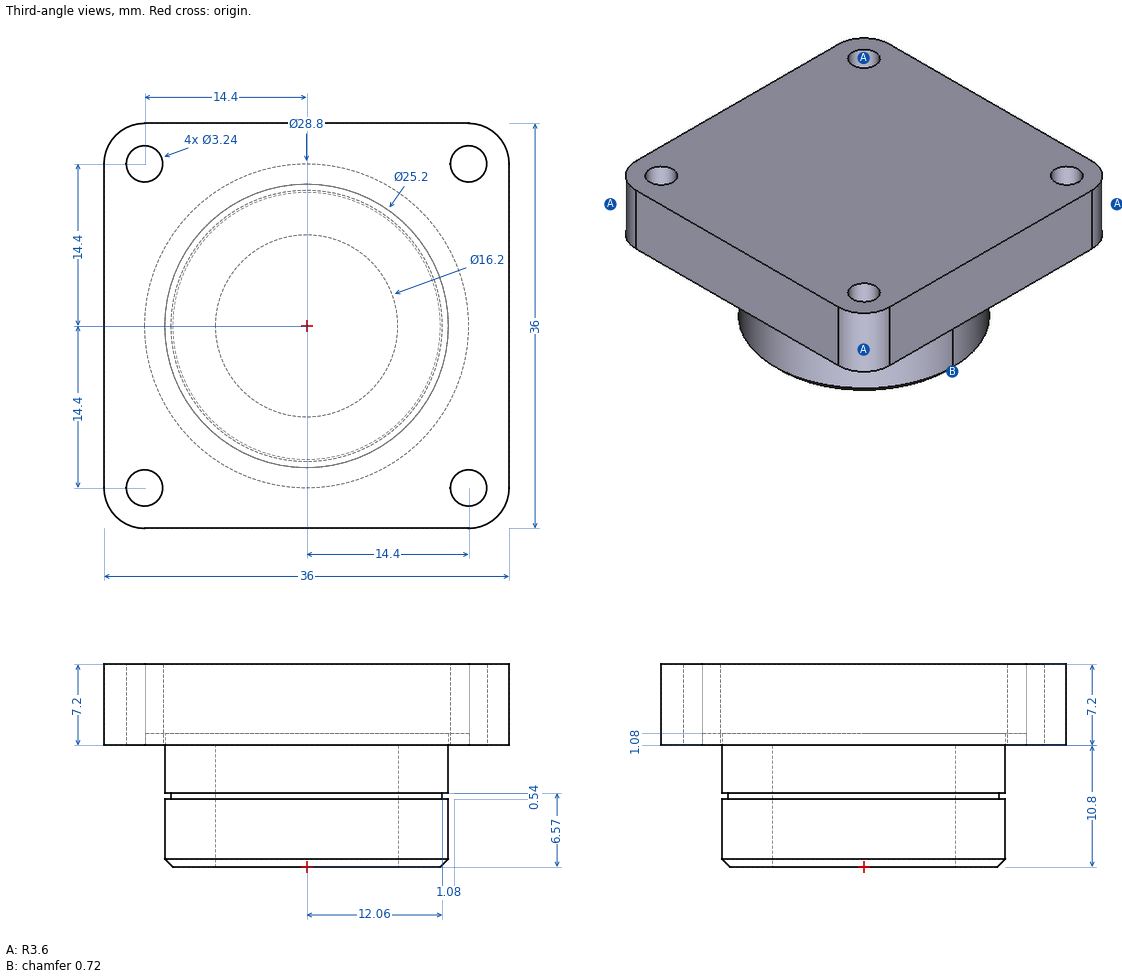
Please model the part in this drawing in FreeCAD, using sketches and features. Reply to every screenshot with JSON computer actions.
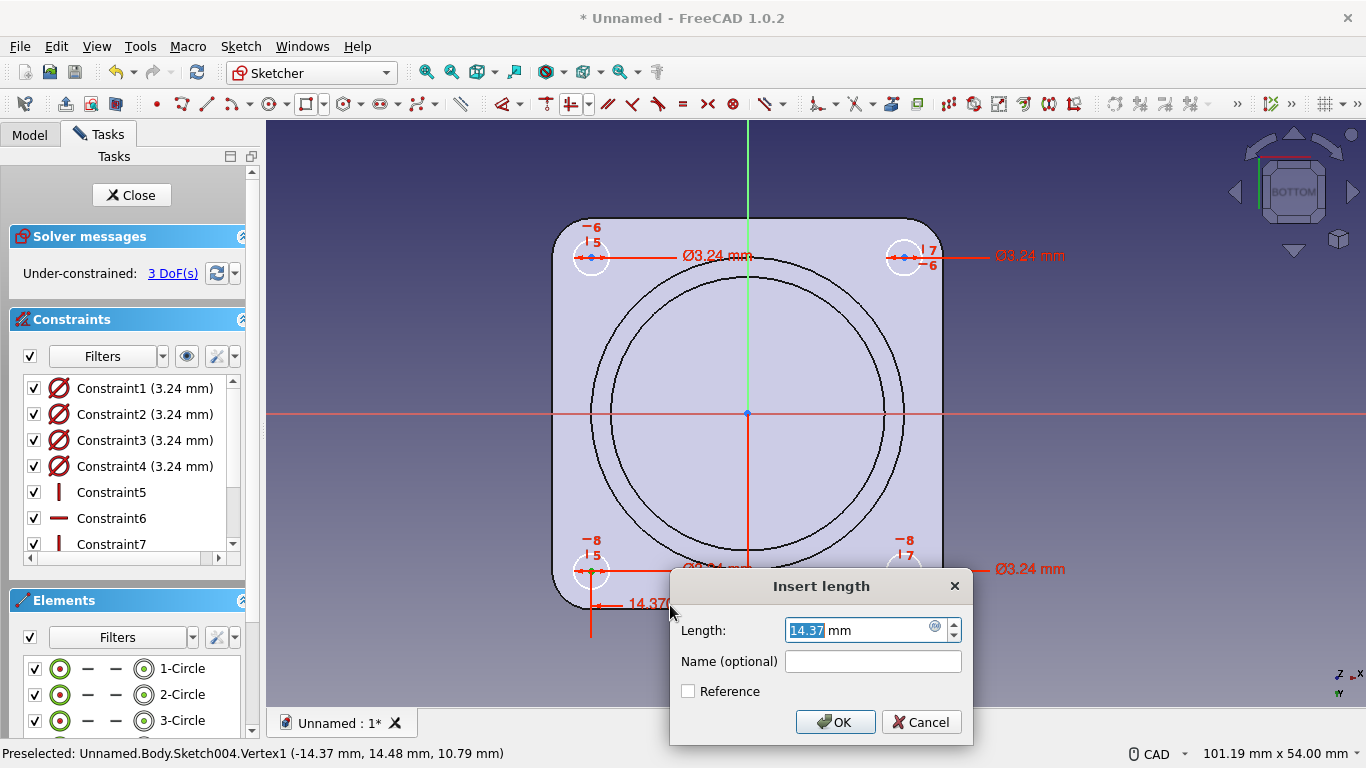
{"action": "type", "text": "14.4"}
{"action": "key", "text": "Return"}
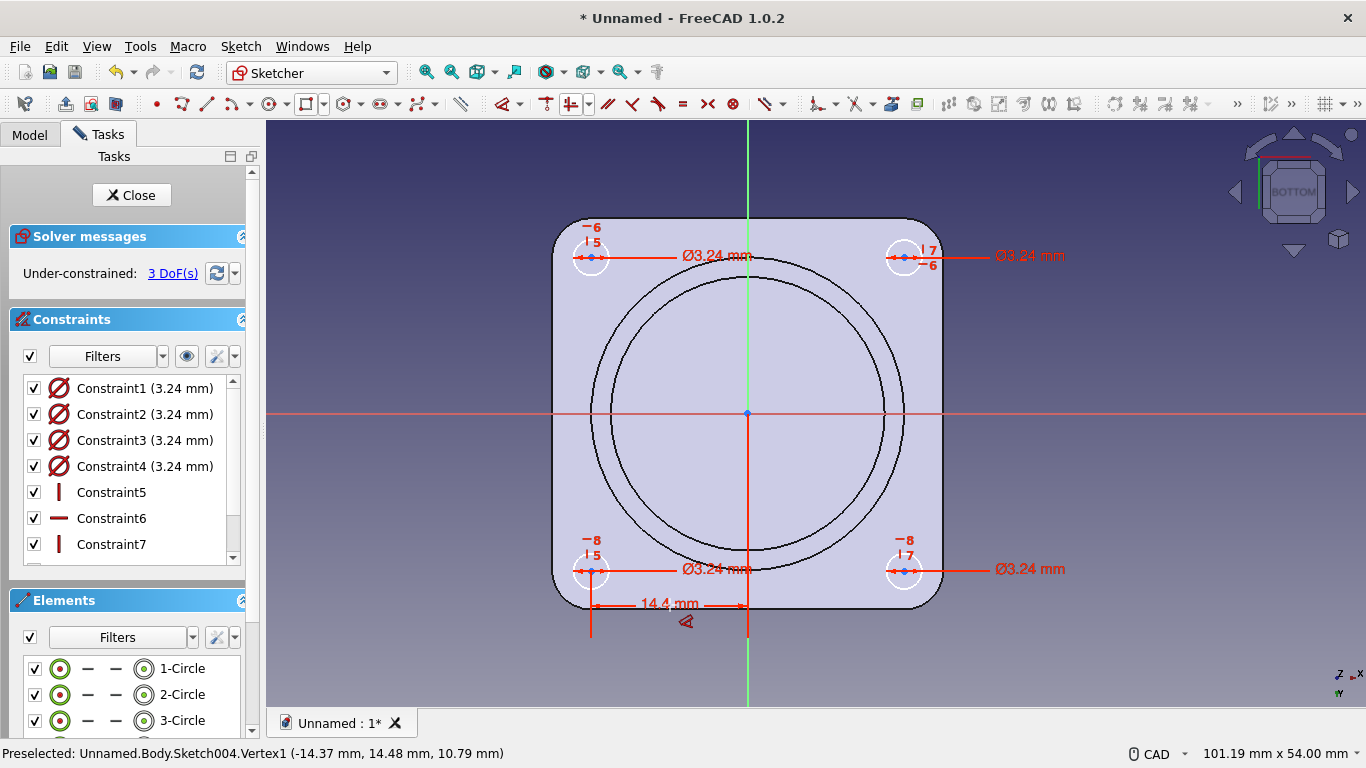
{"action": "left_click", "coordinate": [591, 571]}
{"action": "left_click", "coordinate": [557, 493]}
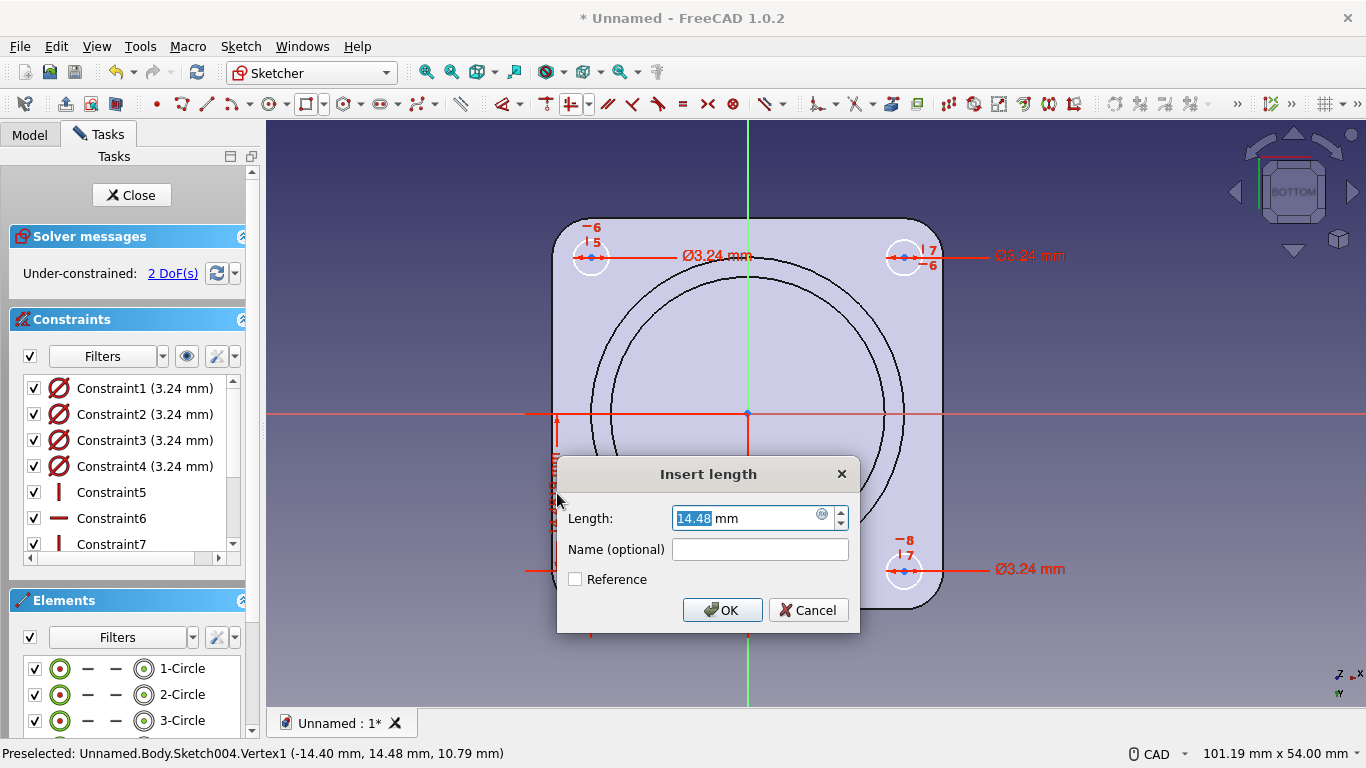
{"action": "type", "text": "14.4"}
{"action": "key", "text": "Return"}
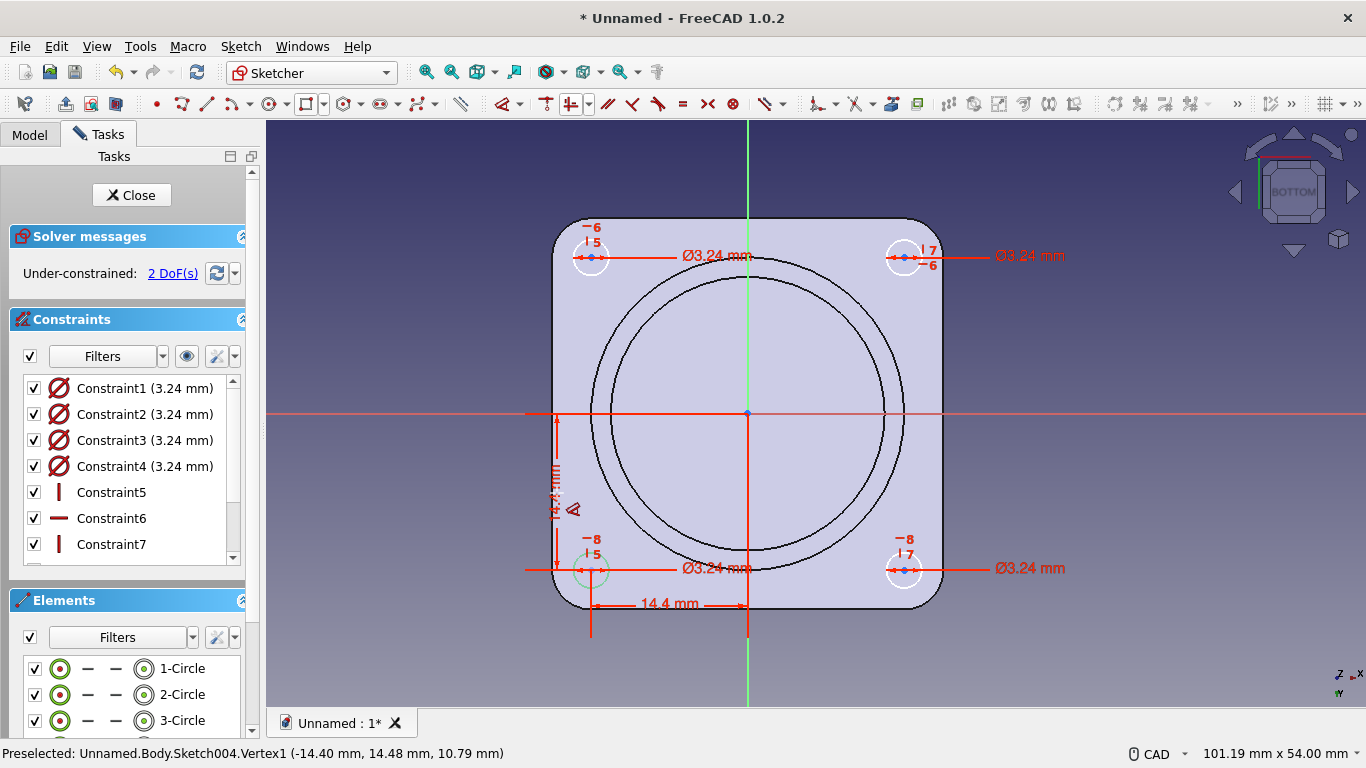
{"action": "left_click", "coordinate": [591, 258]}
{"action": "left_click", "coordinate": [557, 336]}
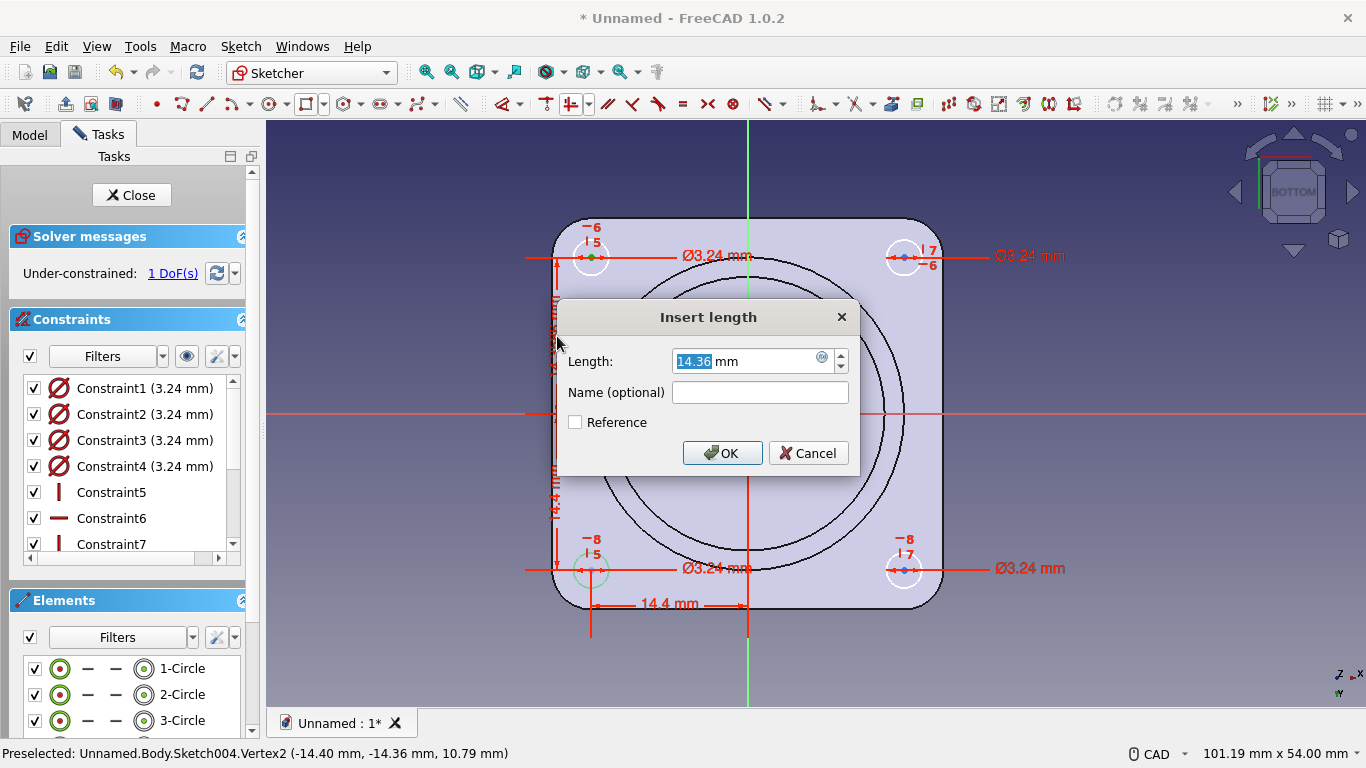
{"action": "type", "text": "14.4"}
{"action": "key", "text": "Return"}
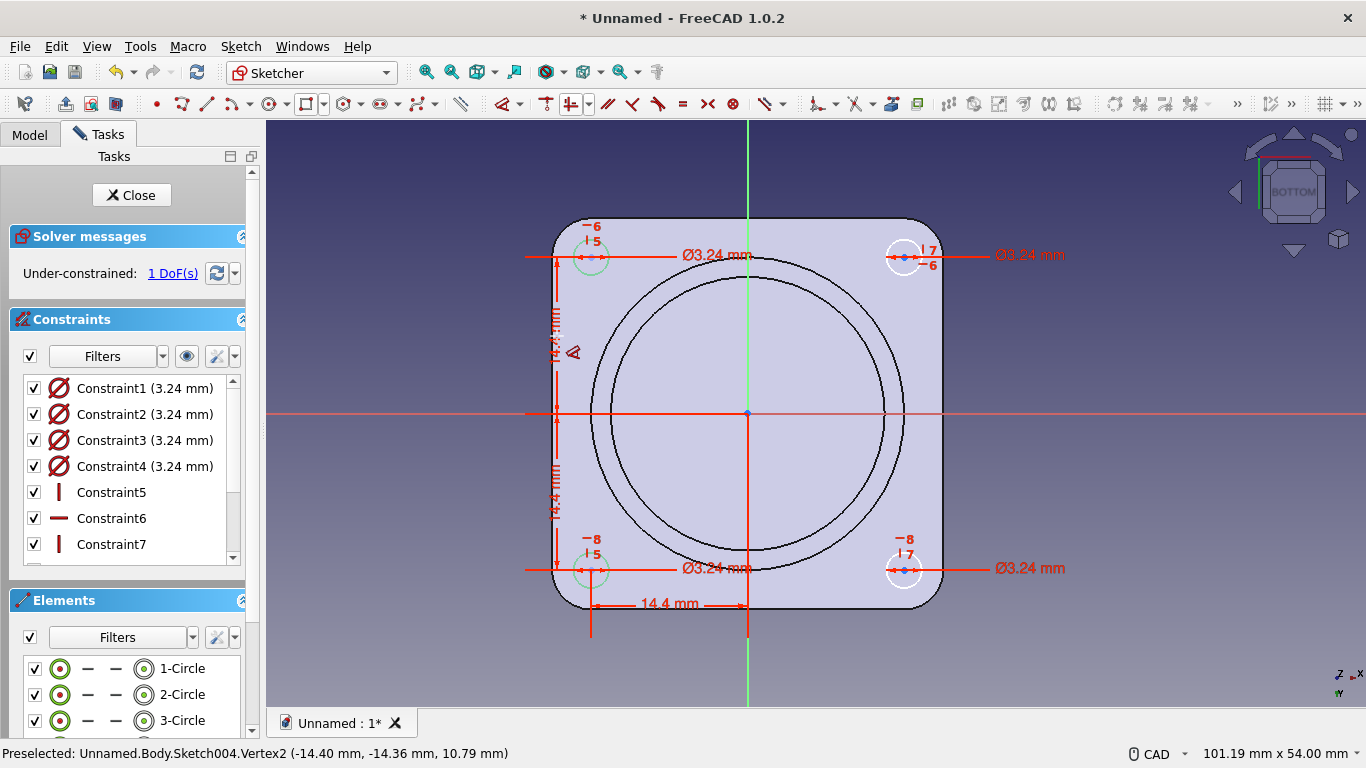
{"action": "left_click", "coordinate": [904, 257]}
{"action": "left_click", "coordinate": [826, 223]}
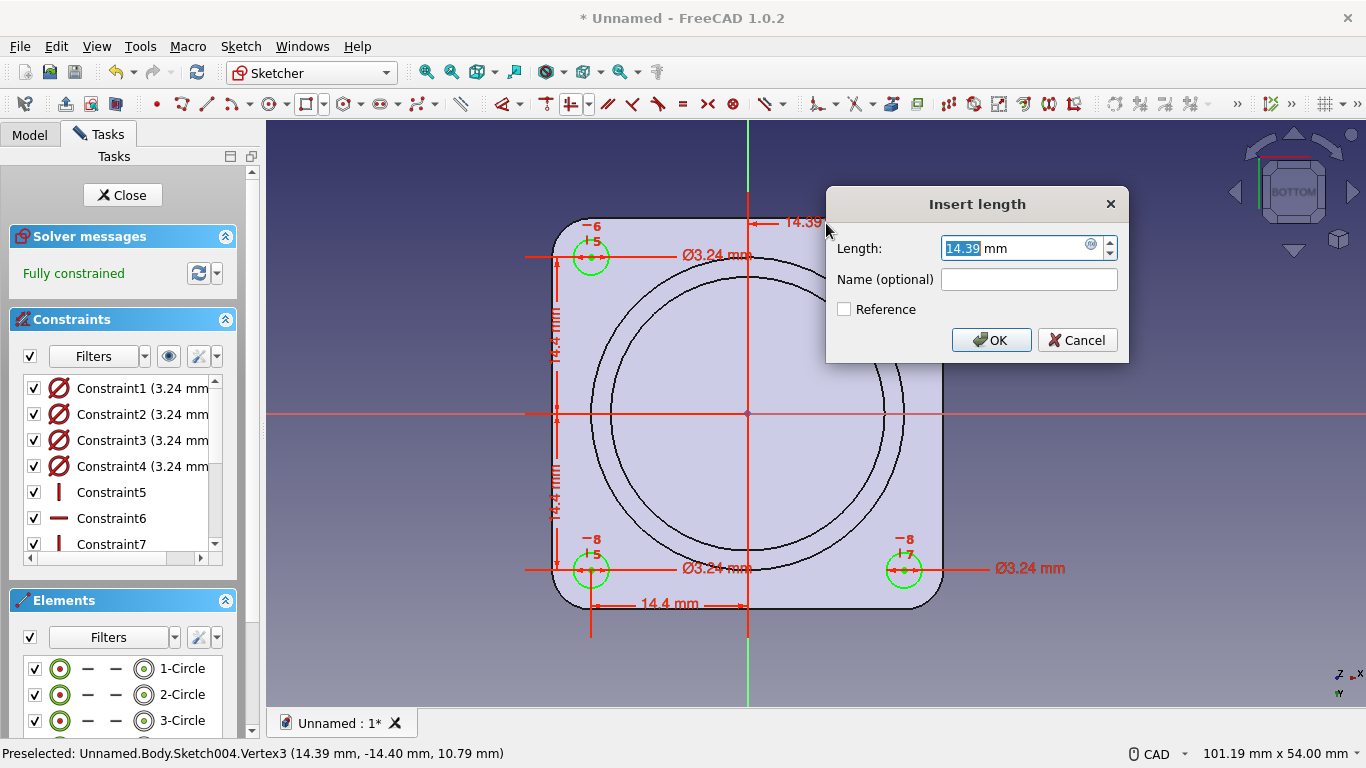
{"action": "type", "text": "14.4"}
{"action": "key", "text": "Return"}
{"action": "key", "text": "Escape"}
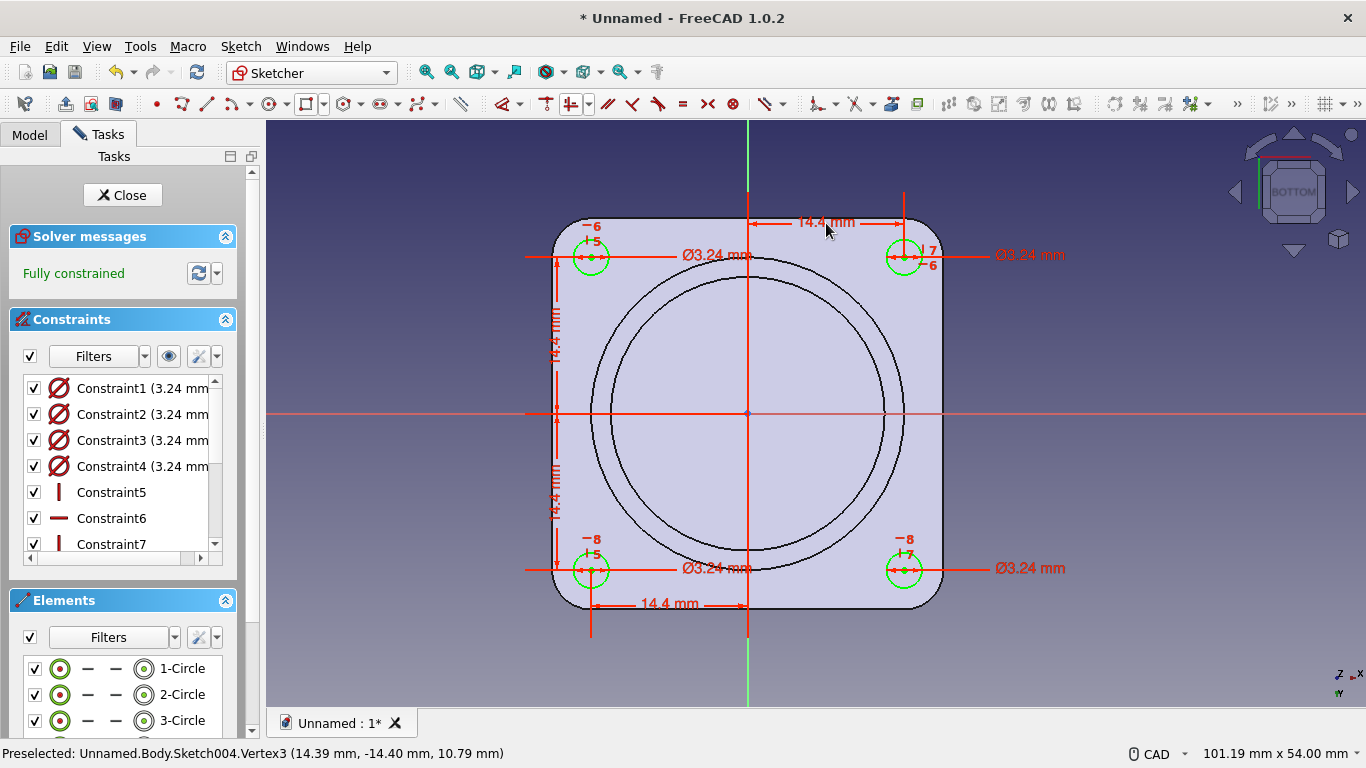
{"action": "left_click", "coordinate": [123, 195]}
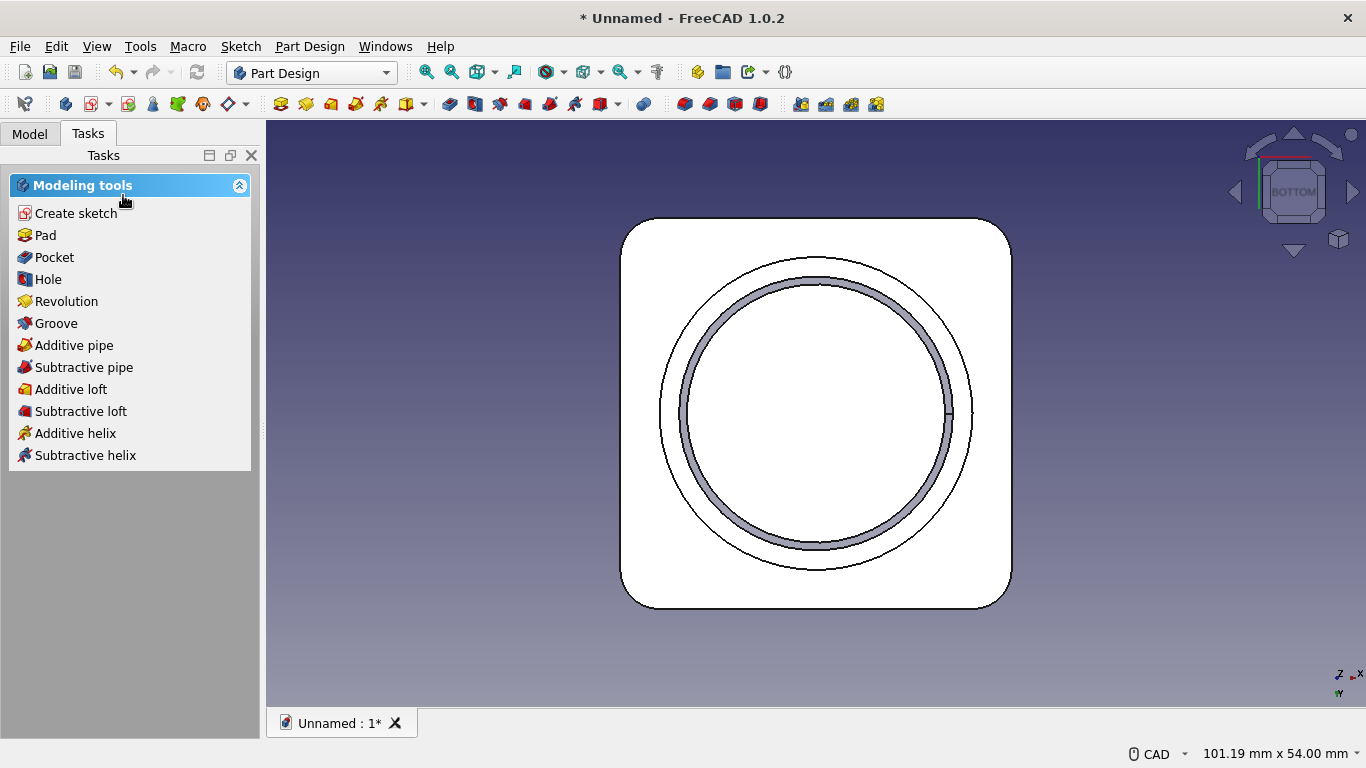
{"action": "left_click", "coordinate": [450, 104]}